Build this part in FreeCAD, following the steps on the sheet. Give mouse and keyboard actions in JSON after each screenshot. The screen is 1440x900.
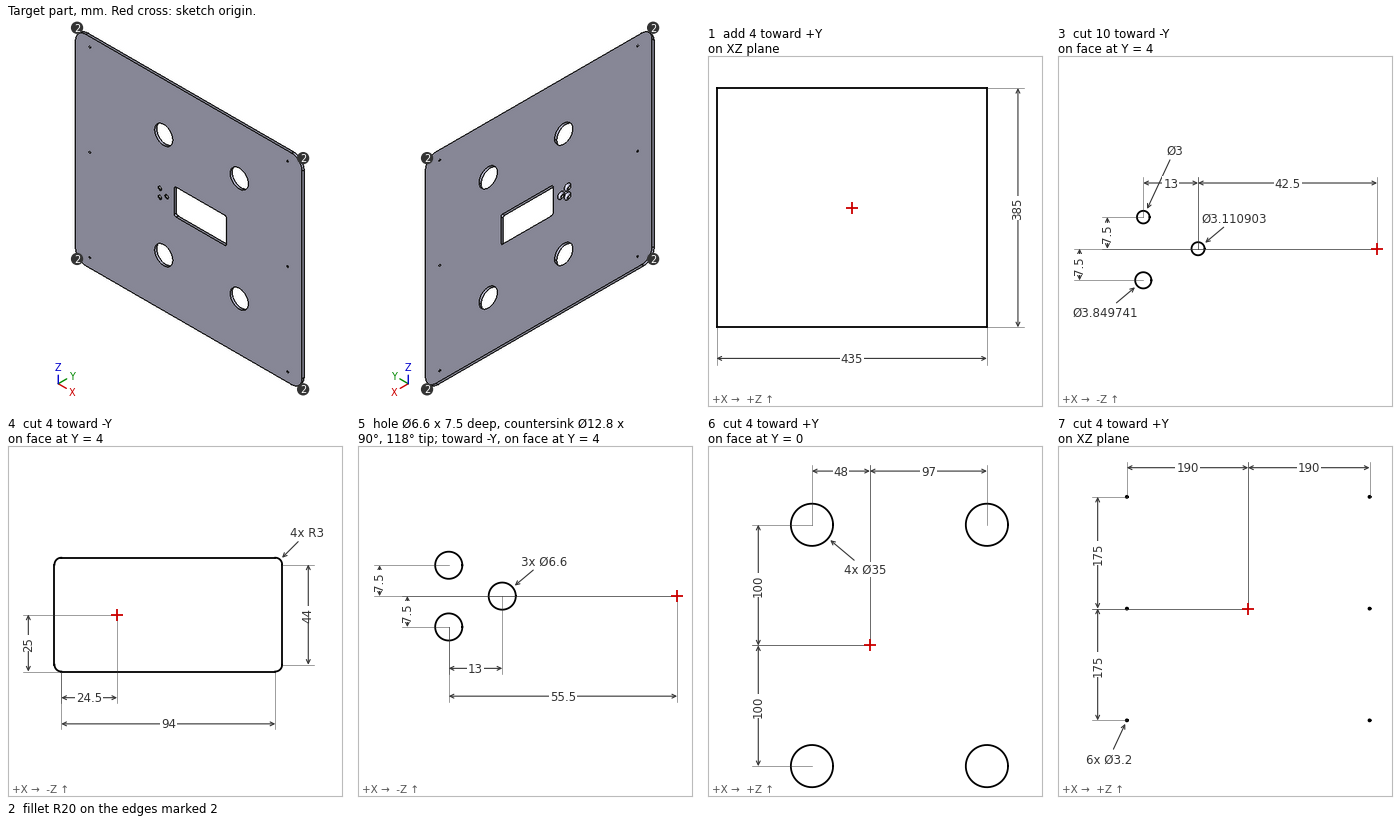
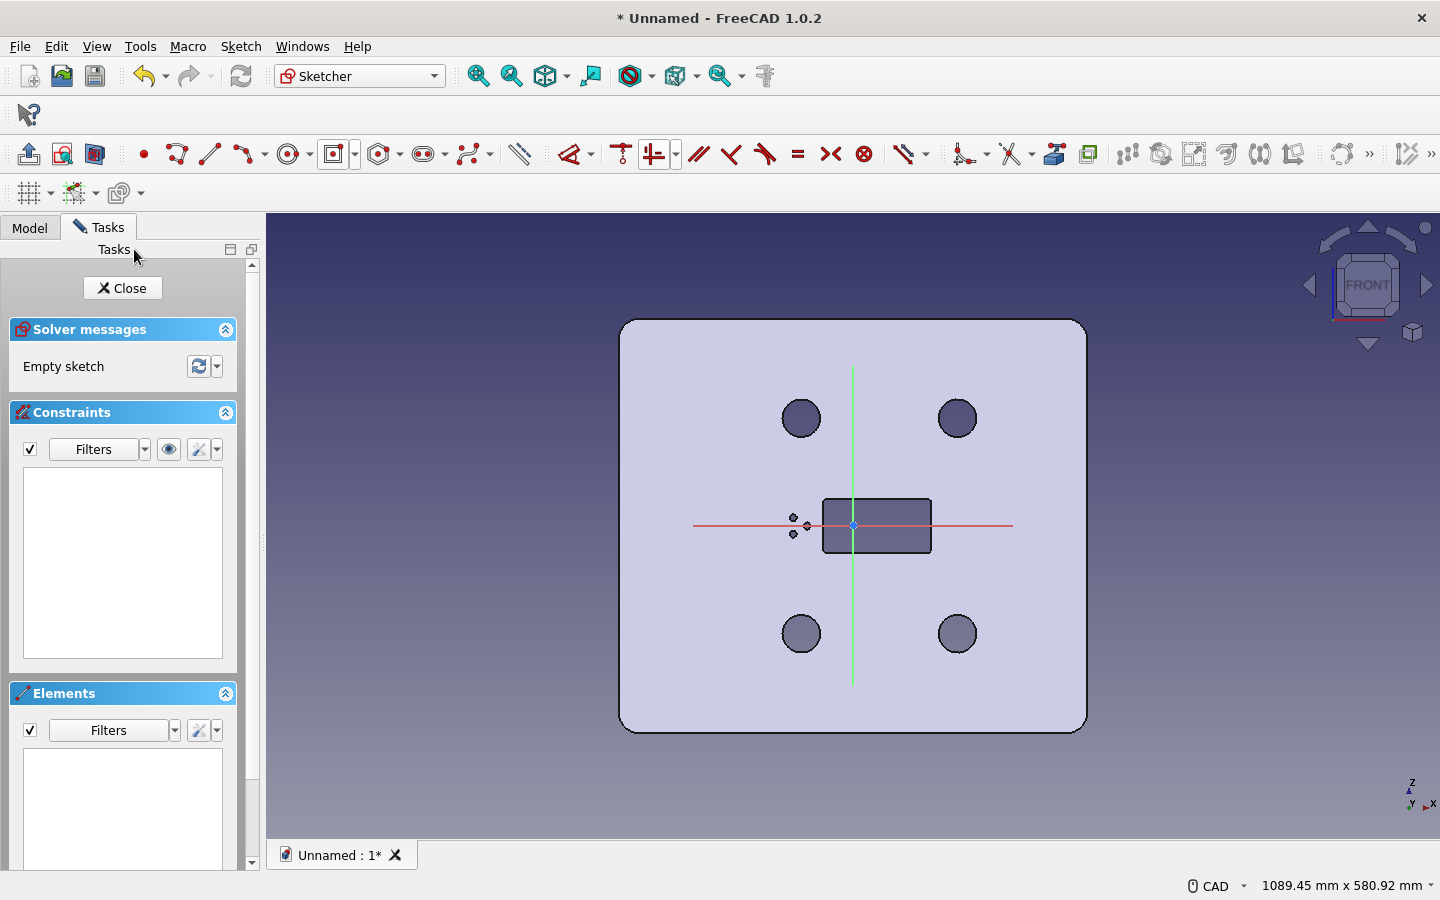
{"action": "left_click", "coordinate": [288, 154]}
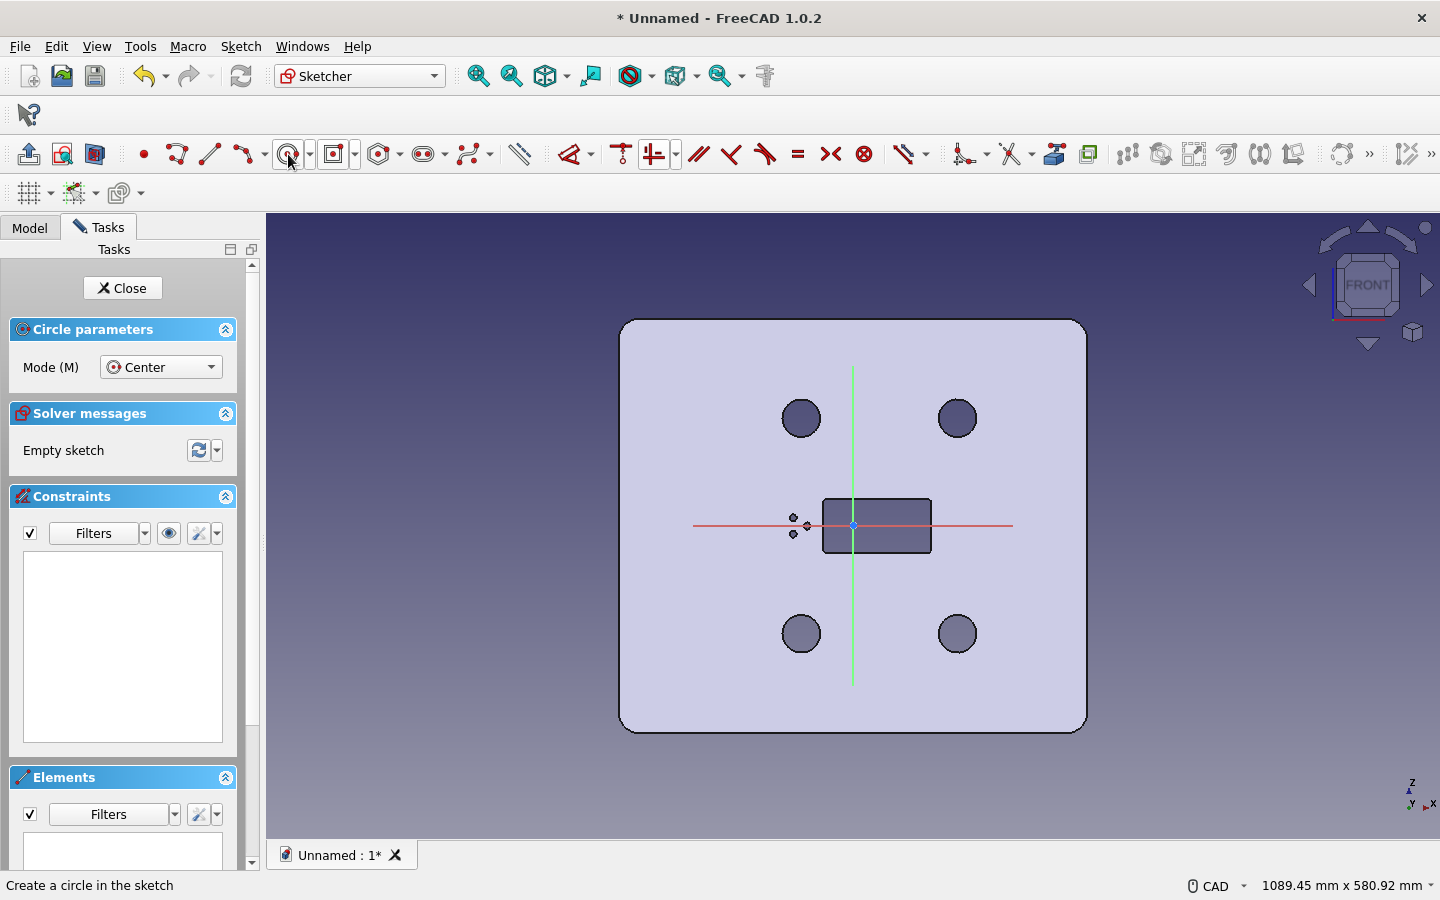
{"action": "scroll", "coordinate": [648, 337], "scroll_direction": "up", "scroll_amount": 13}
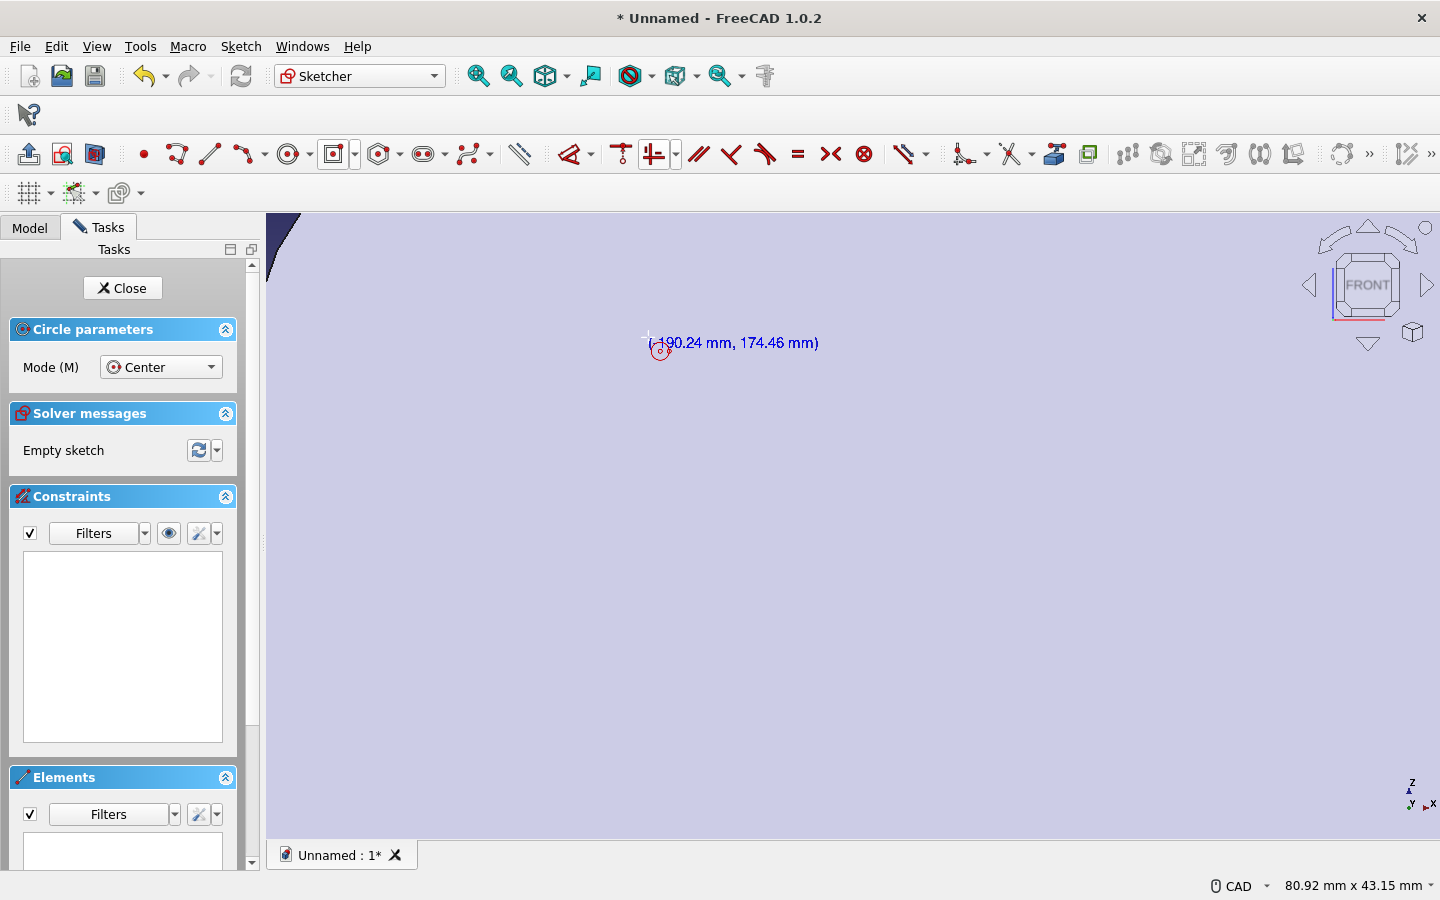
{"action": "scroll", "coordinate": [574, 337], "scroll_direction": "down", "scroll_amount": 13}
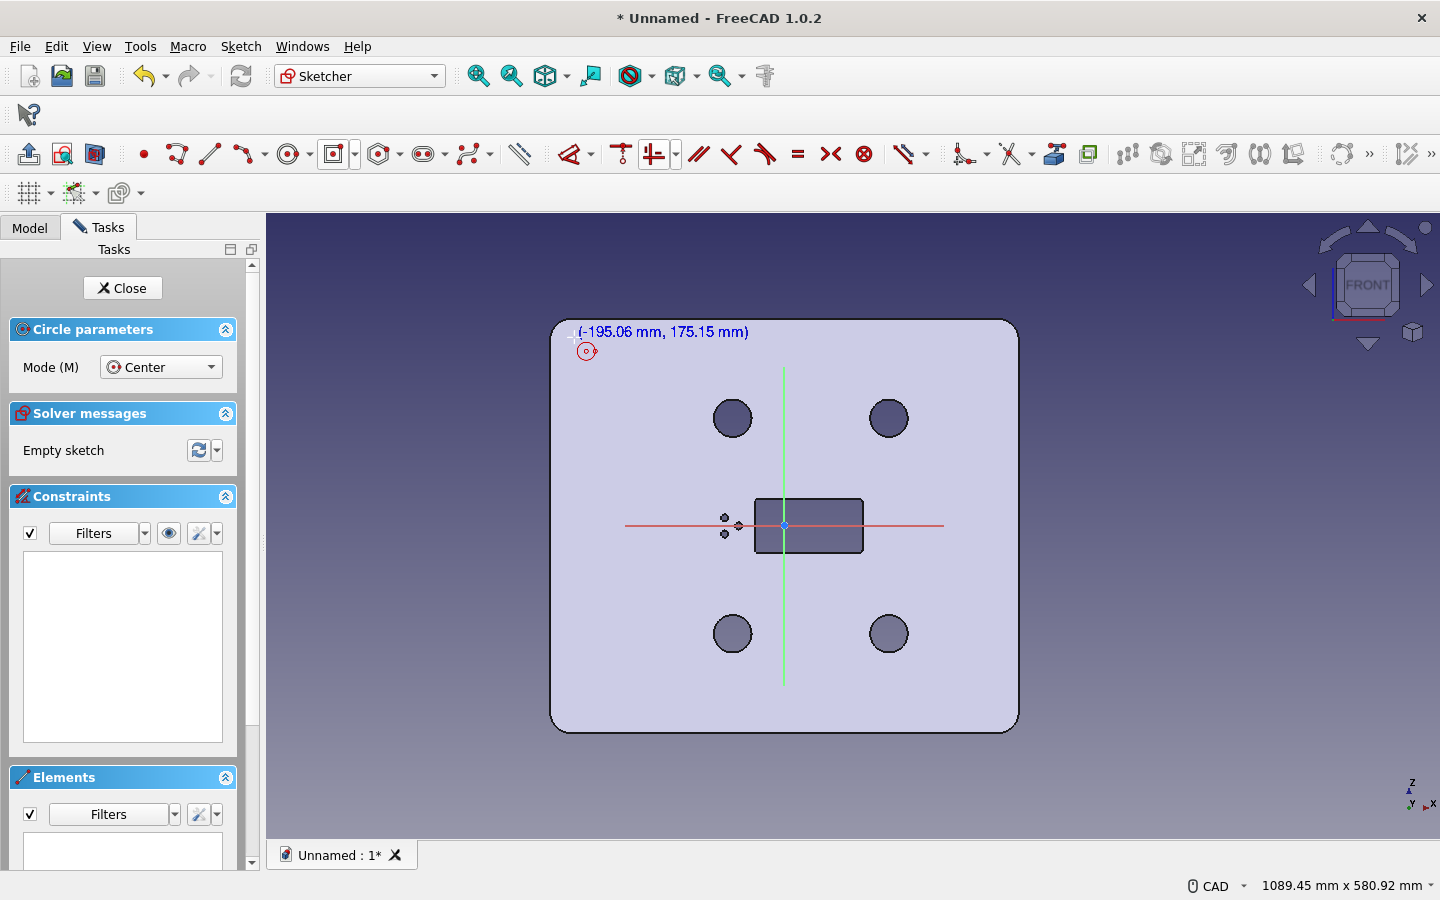
{"action": "left_click", "coordinate": [580, 337]}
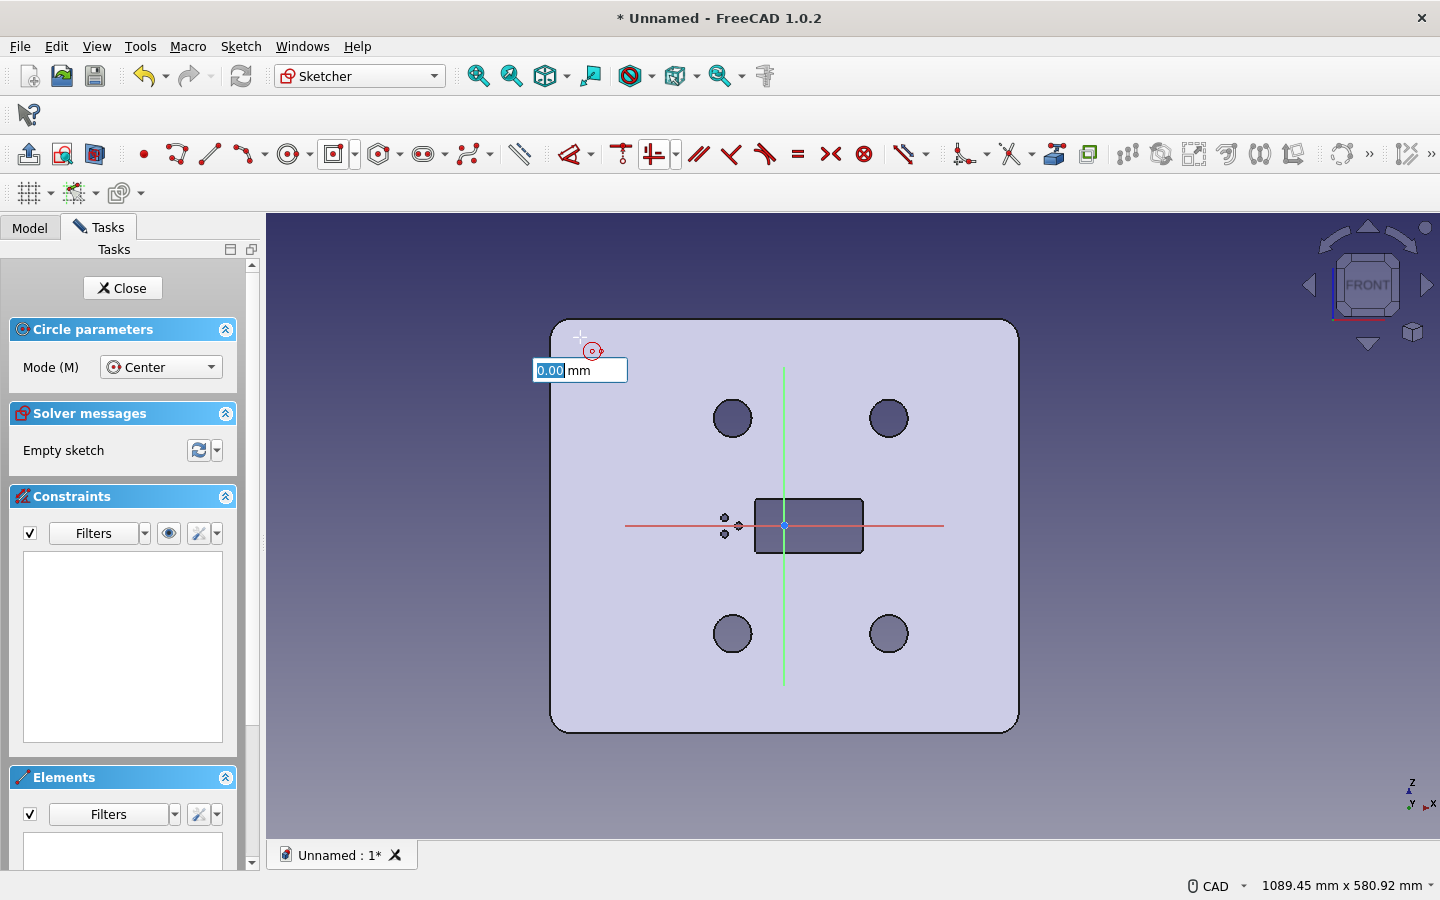
{"action": "scroll", "coordinate": [581, 336], "scroll_direction": "up", "scroll_amount": 12}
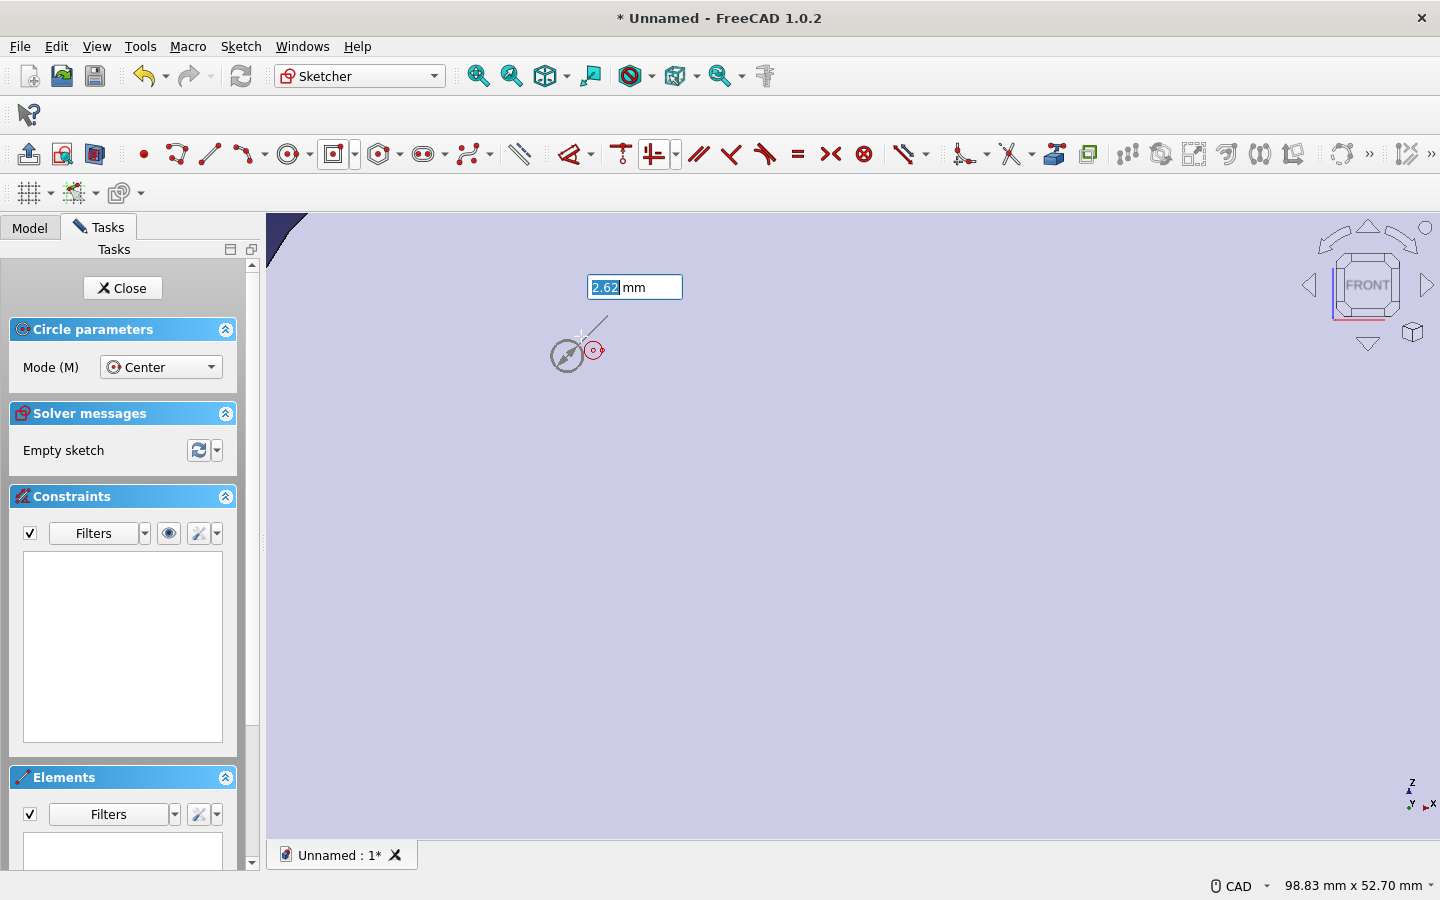
{"action": "left_click", "coordinate": [577, 336]}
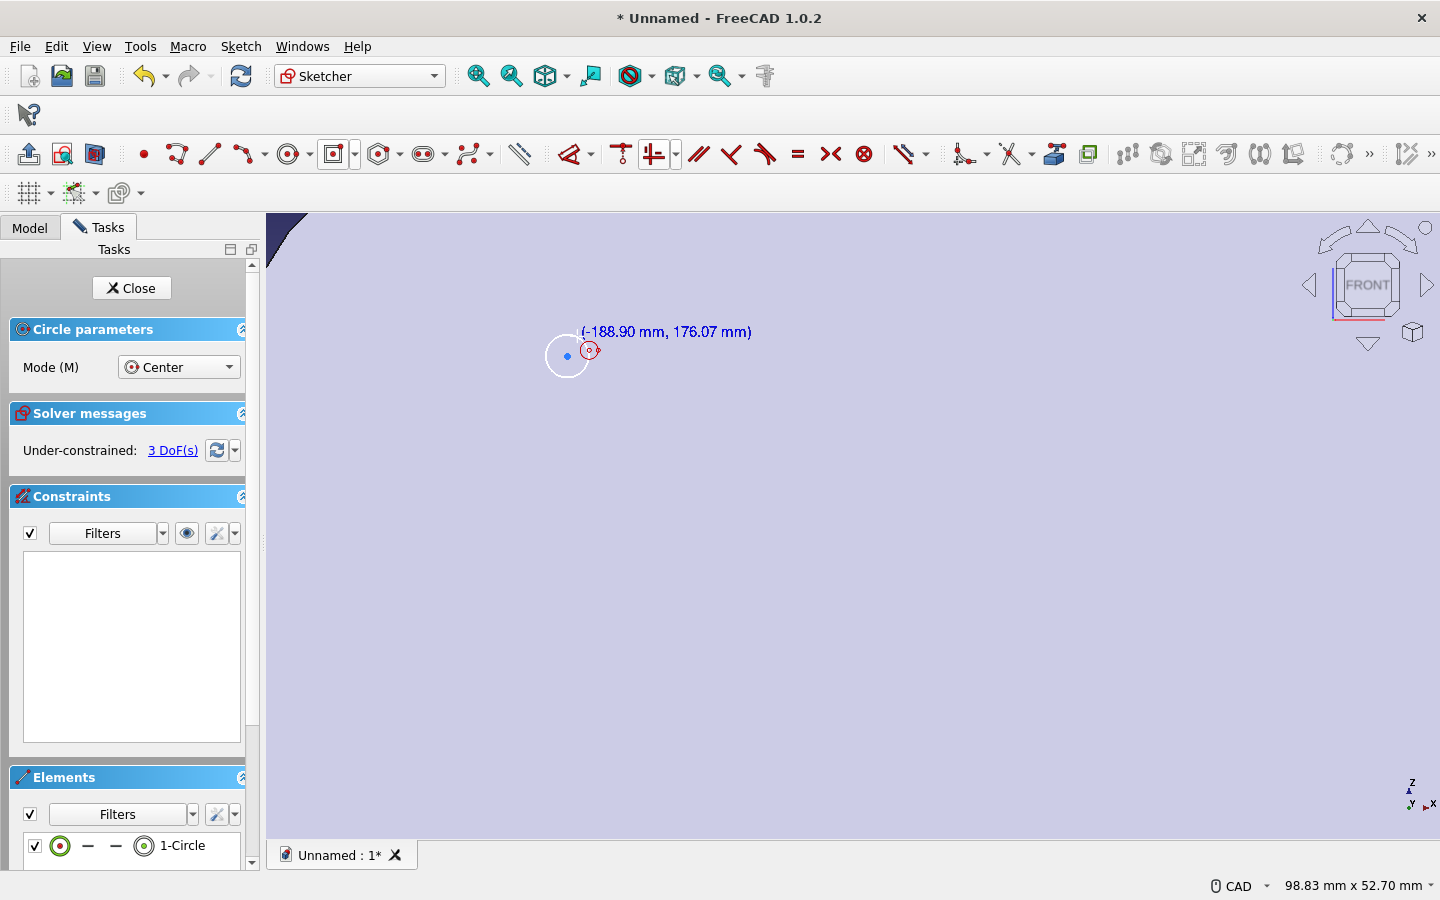
{"action": "scroll", "coordinate": [581, 336], "scroll_direction": "down", "scroll_amount": 12}